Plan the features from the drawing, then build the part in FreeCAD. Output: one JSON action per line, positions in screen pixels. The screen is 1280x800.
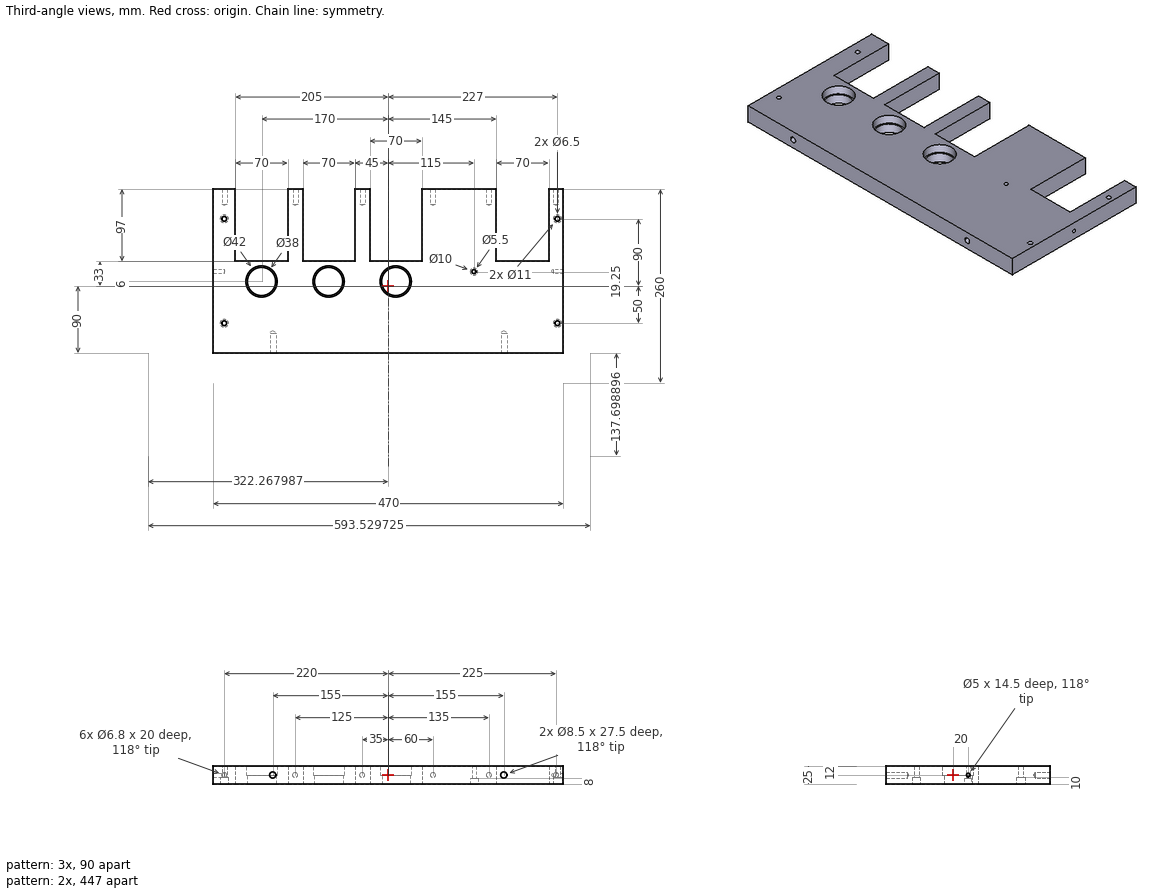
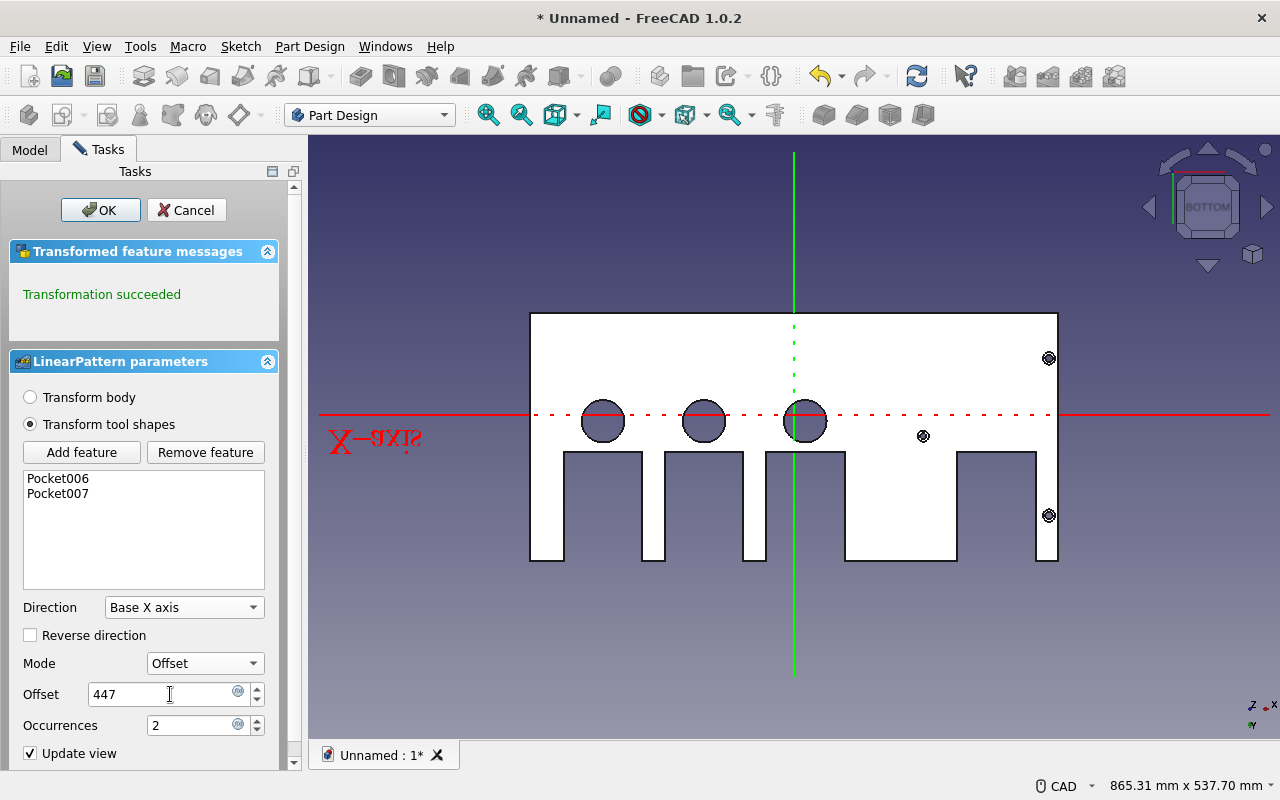
{"action": "triple_click", "coordinate": [199, 726]}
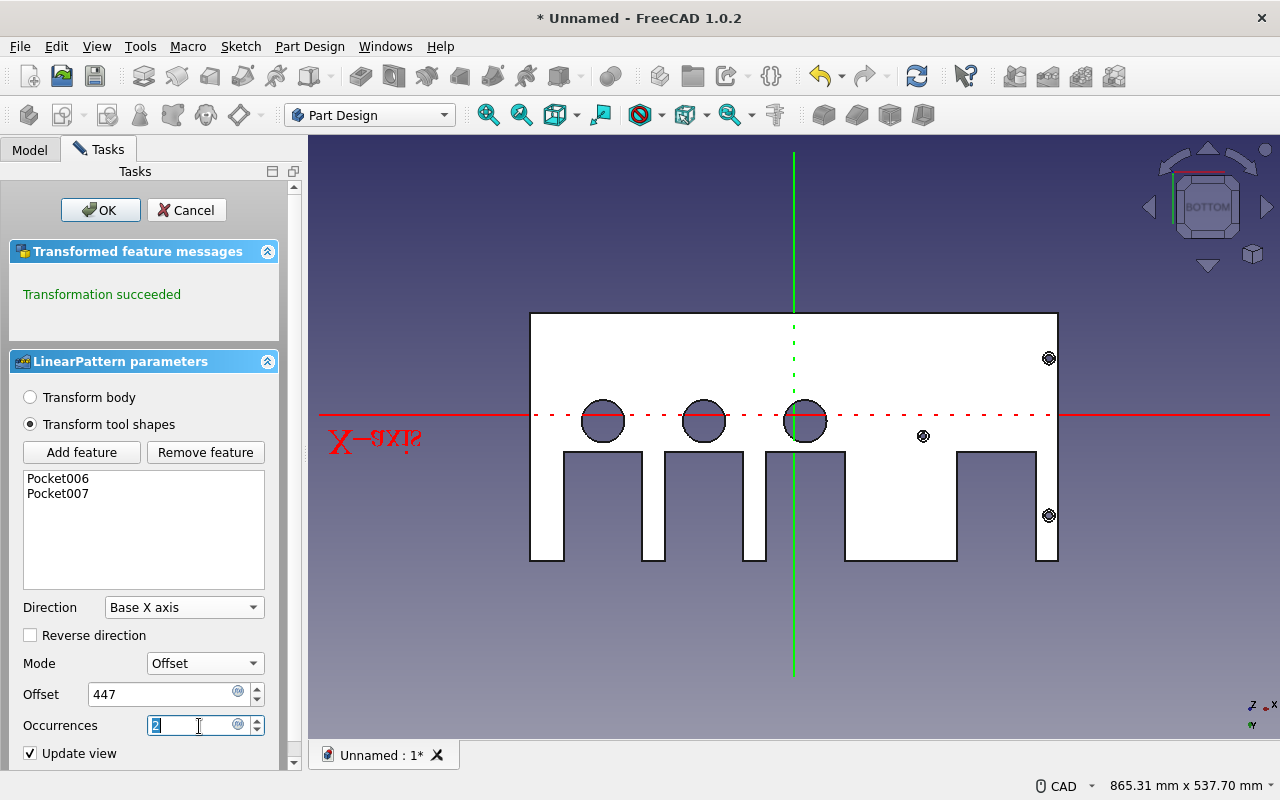
{"action": "type", "text": "2"}
{"action": "key", "text": "Tab"}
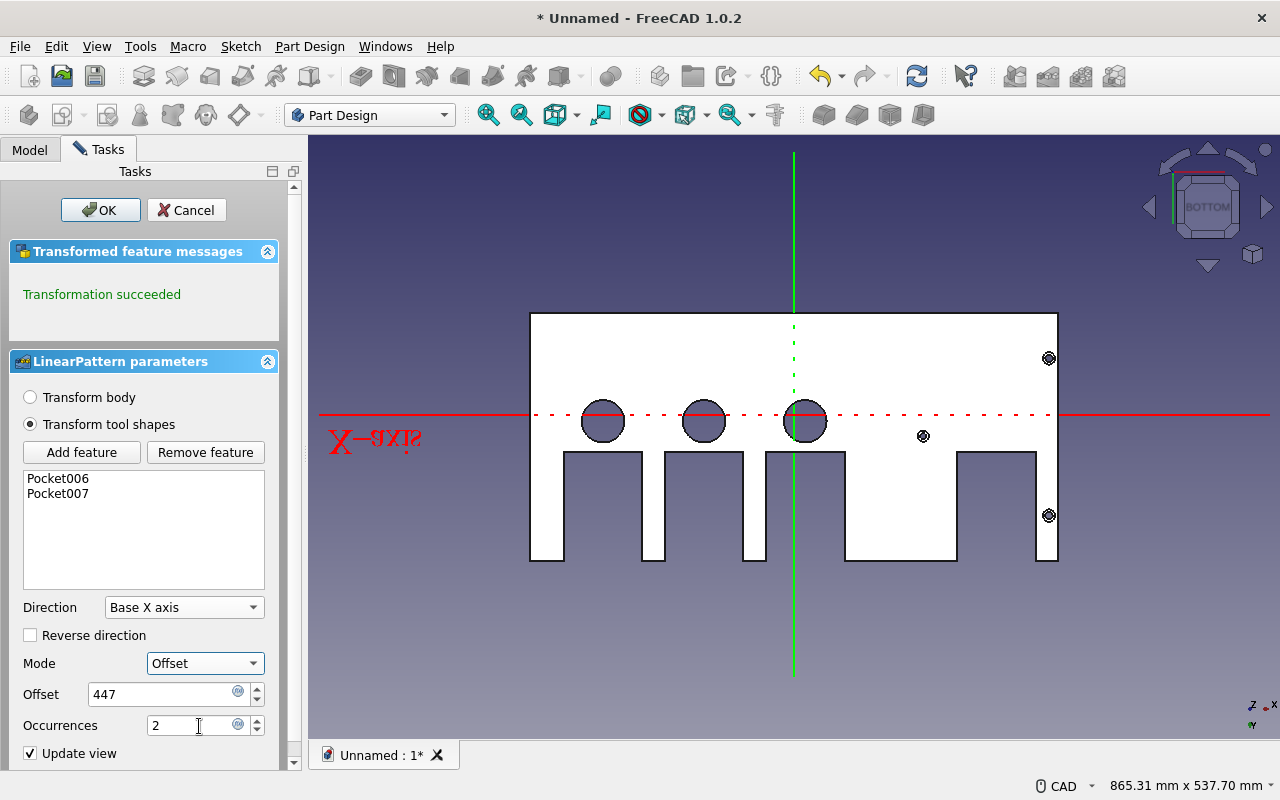
{"action": "left_click", "coordinate": [31, 635]}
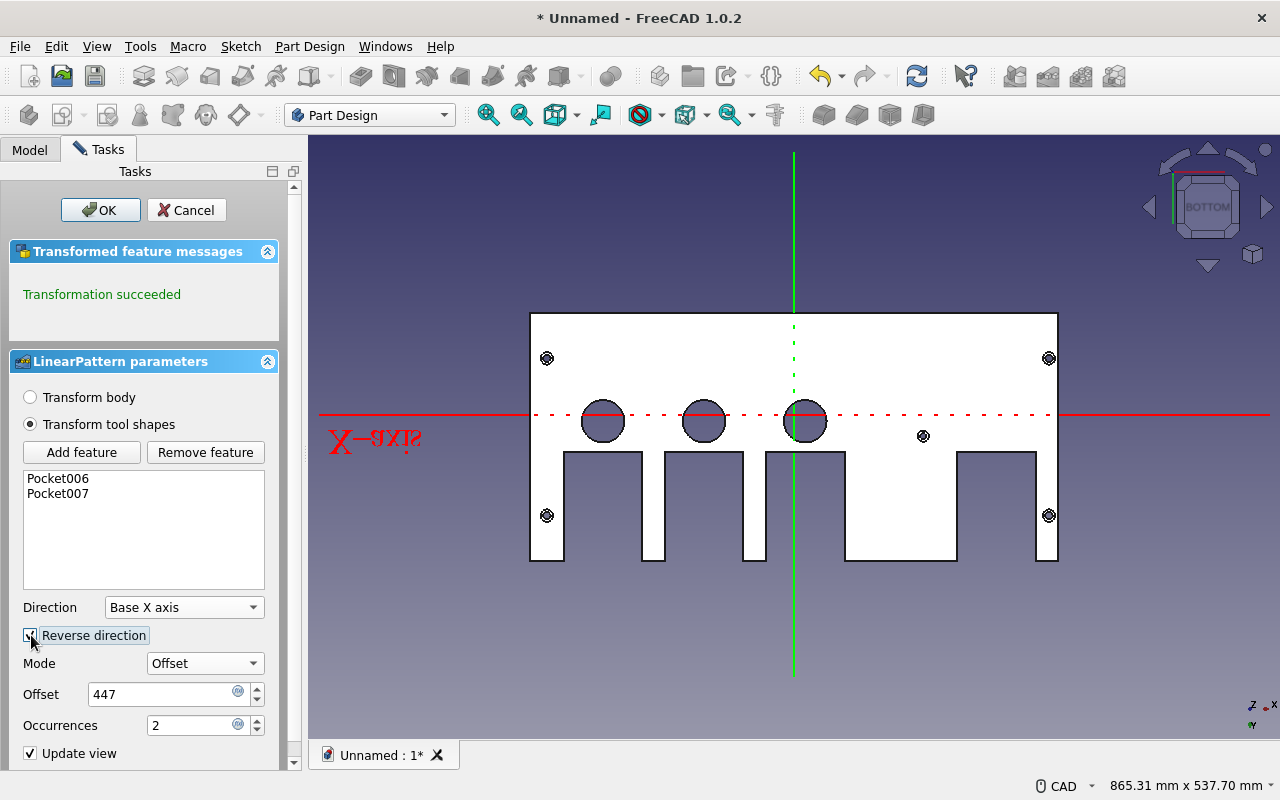
{"action": "left_click", "coordinate": [101, 210]}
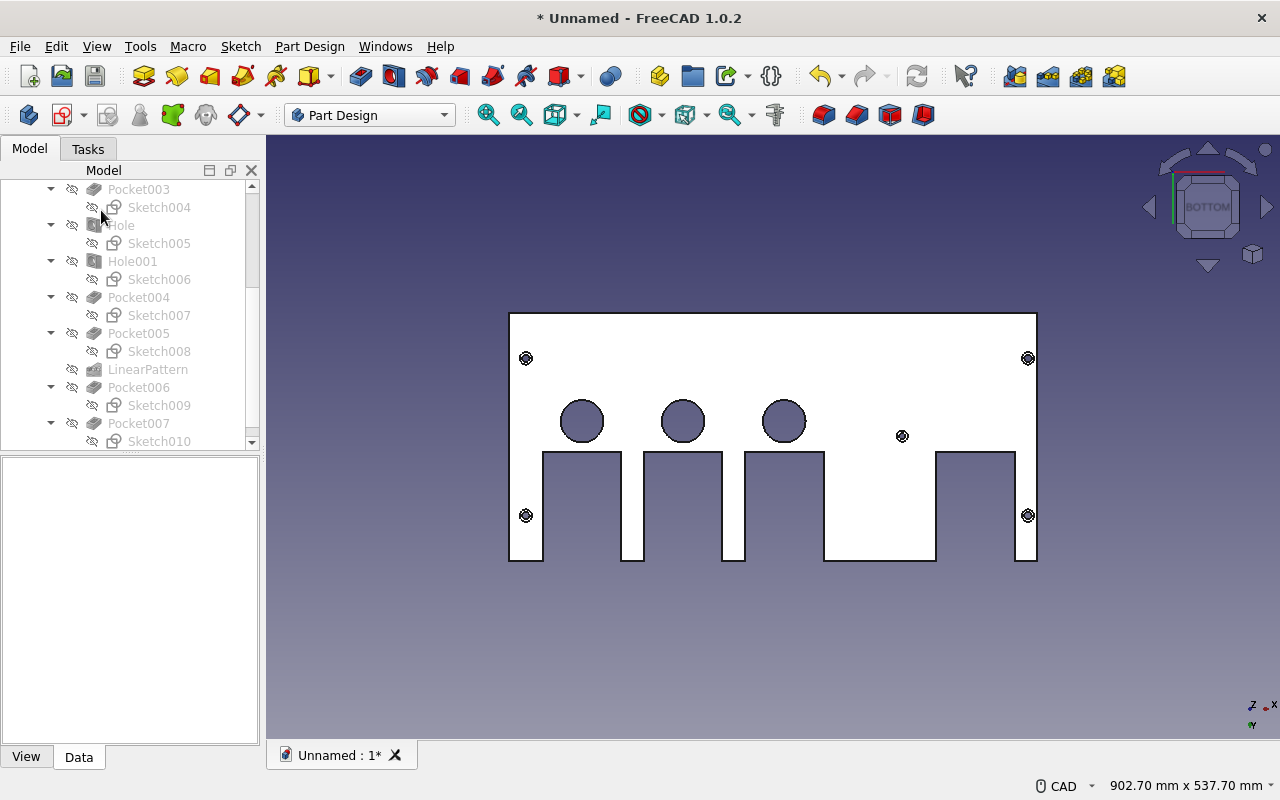
{"action": "key", "text": "6"}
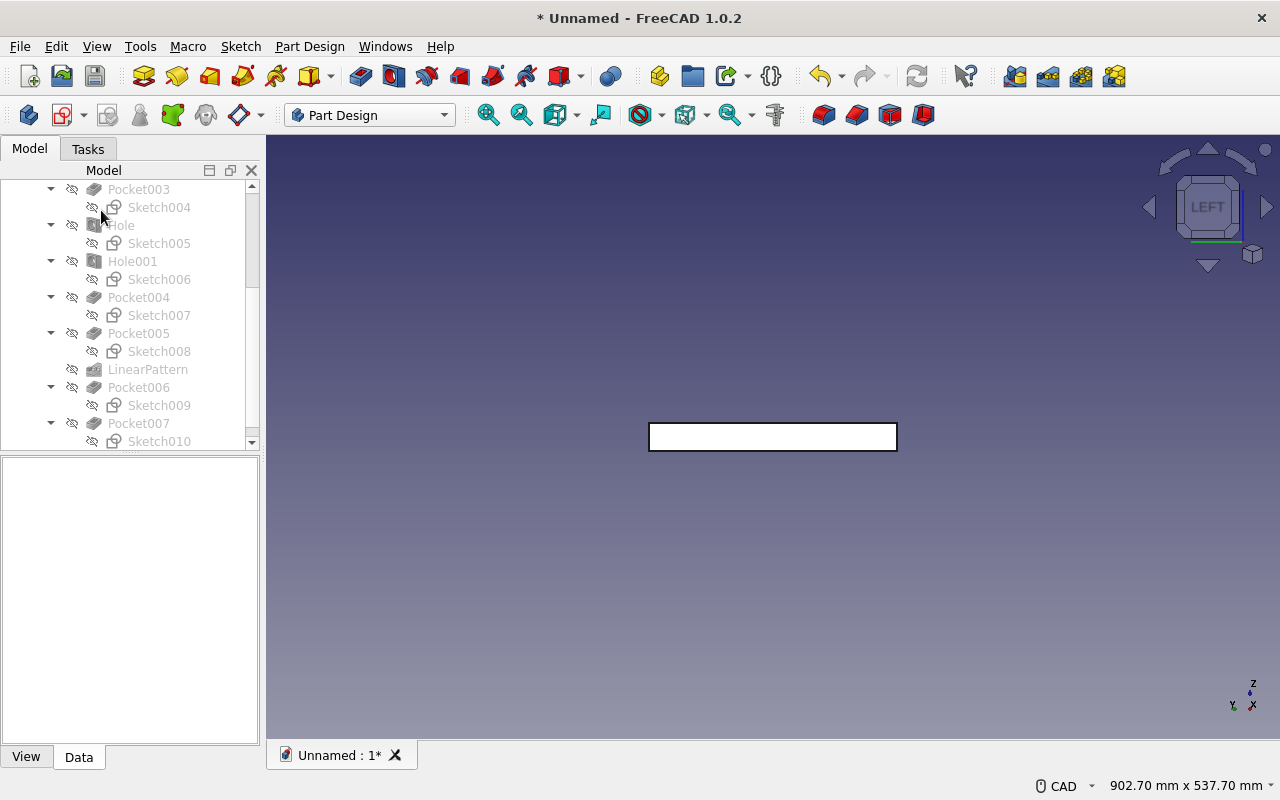
{"action": "left_click", "coordinate": [489, 116]}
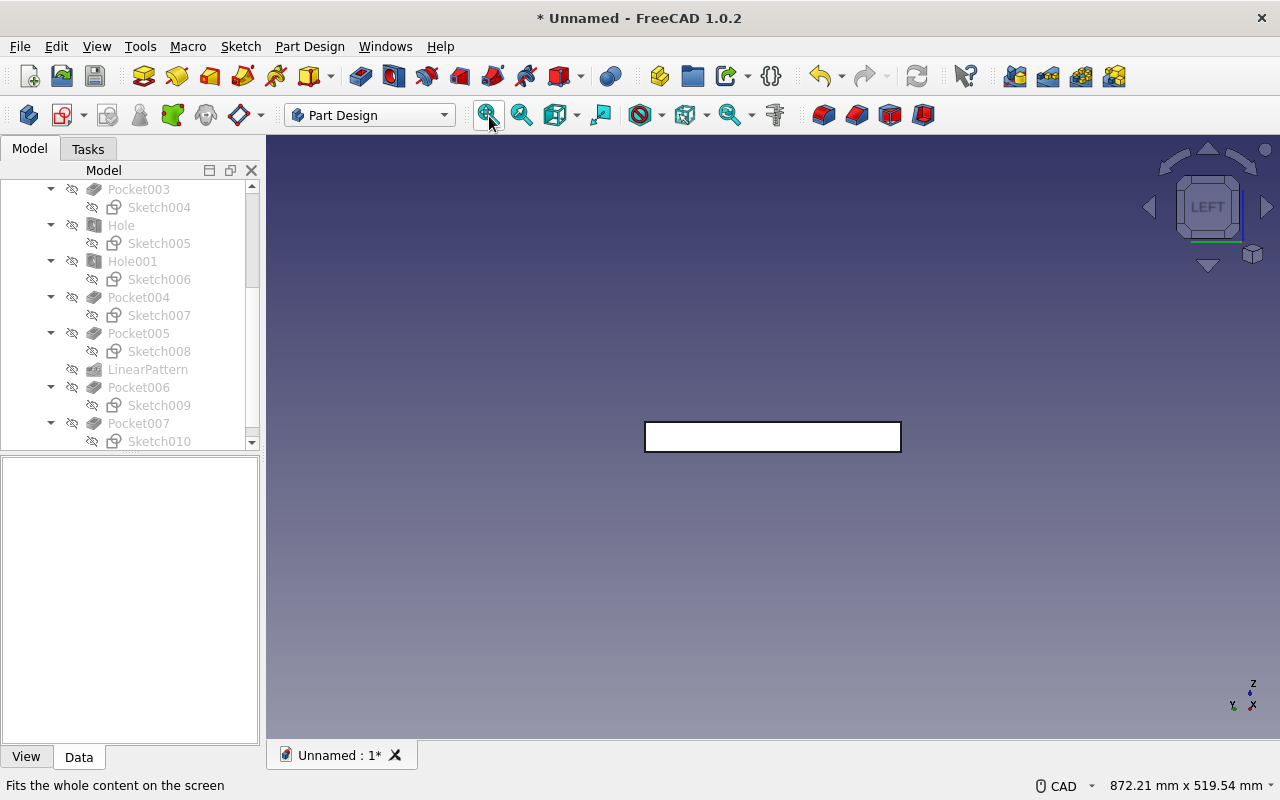
{"action": "left_click", "coordinate": [663, 436]}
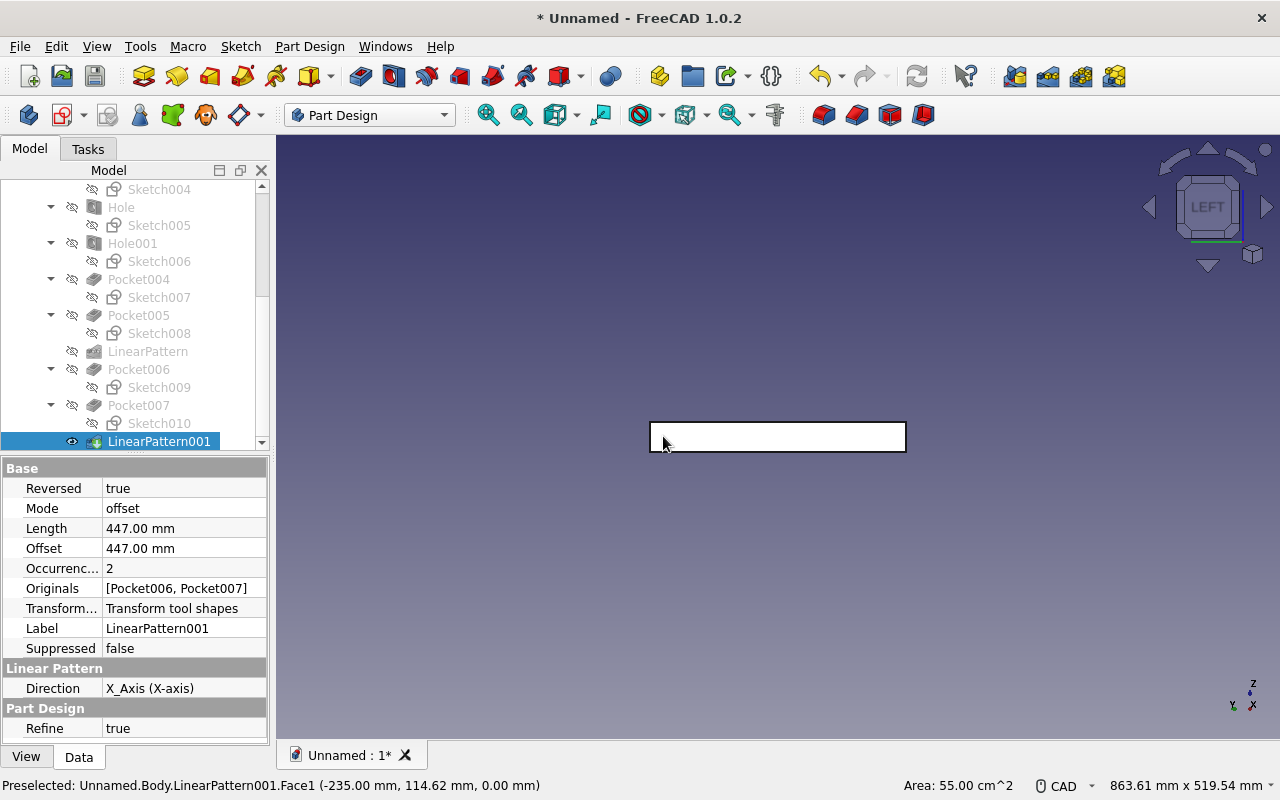
{"action": "left_click", "coordinate": [62, 116]}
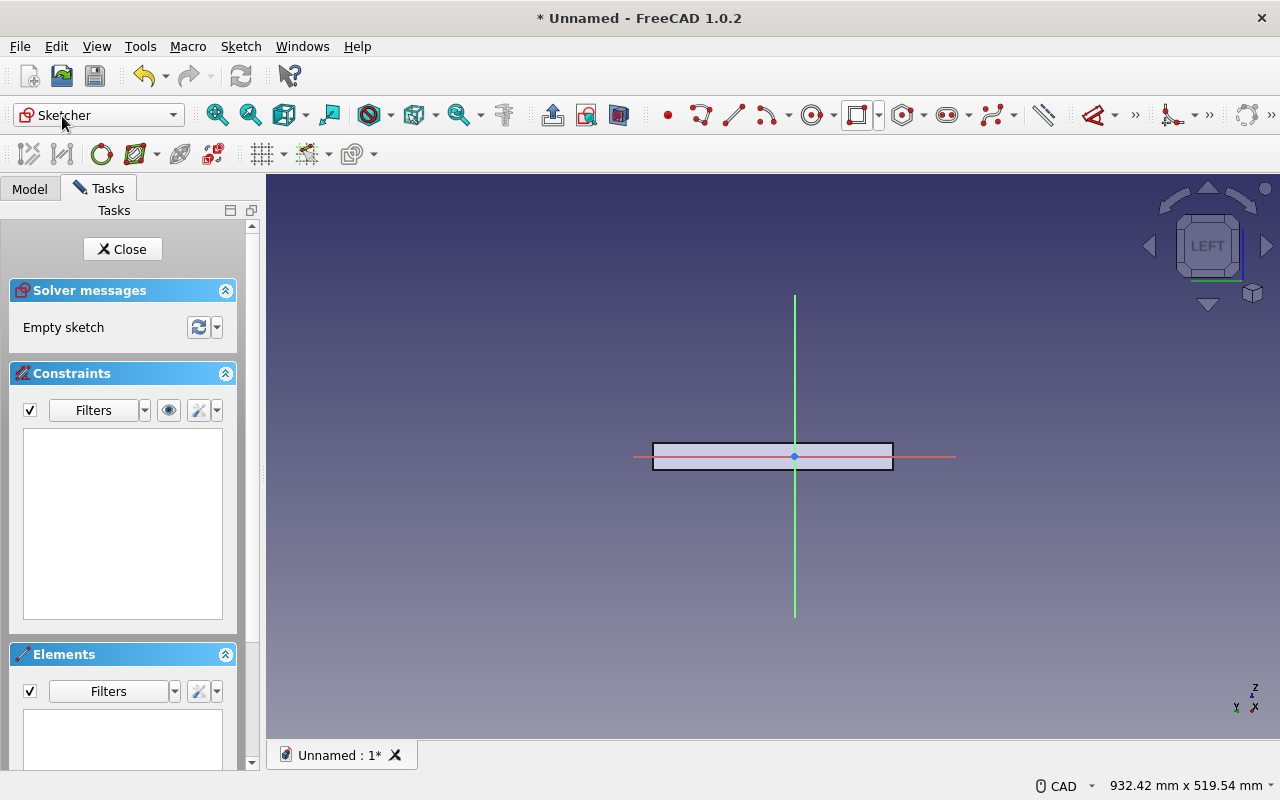
{"action": "scroll", "coordinate": [777, 457], "scroll_direction": "up", "scroll_amount": 15}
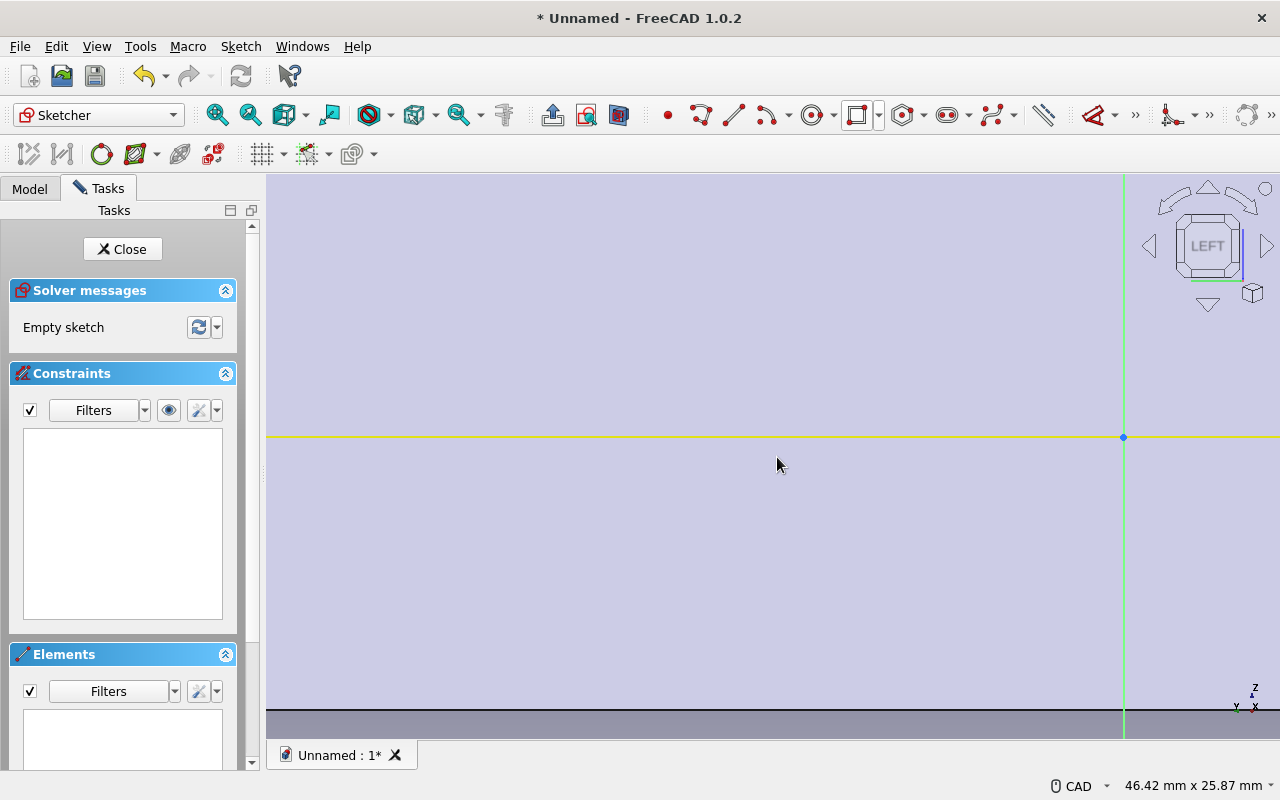
{"action": "scroll", "coordinate": [679, 429], "scroll_direction": "up", "scroll_amount": 6}